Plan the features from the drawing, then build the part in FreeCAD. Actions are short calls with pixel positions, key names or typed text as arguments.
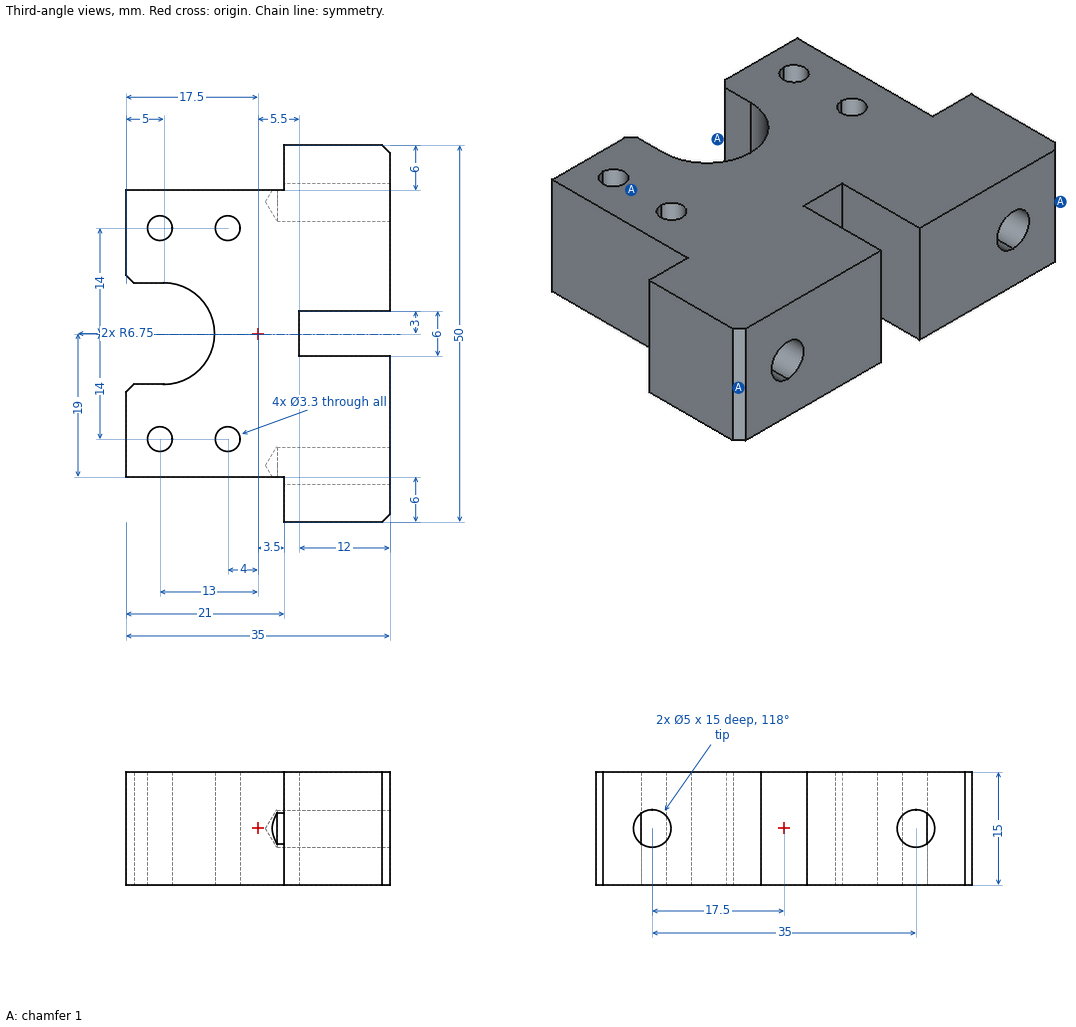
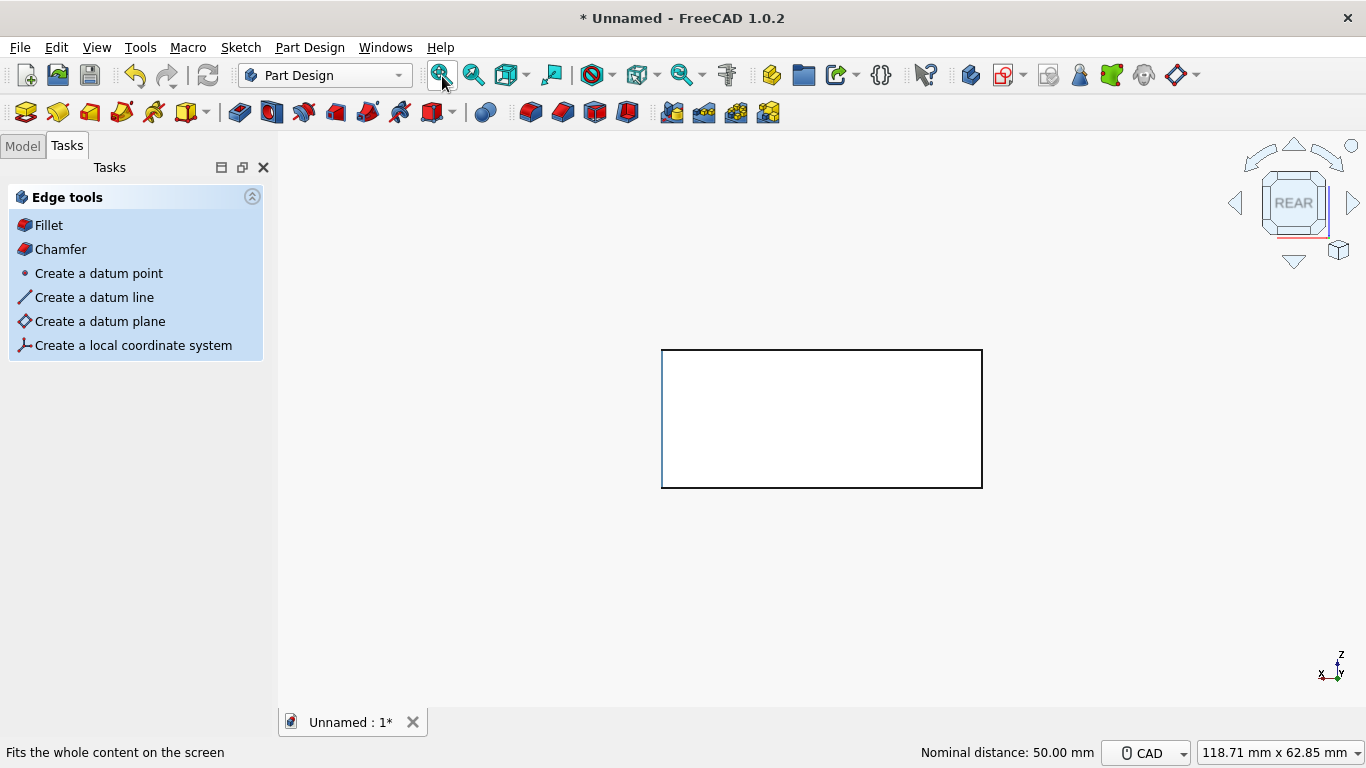
key(6)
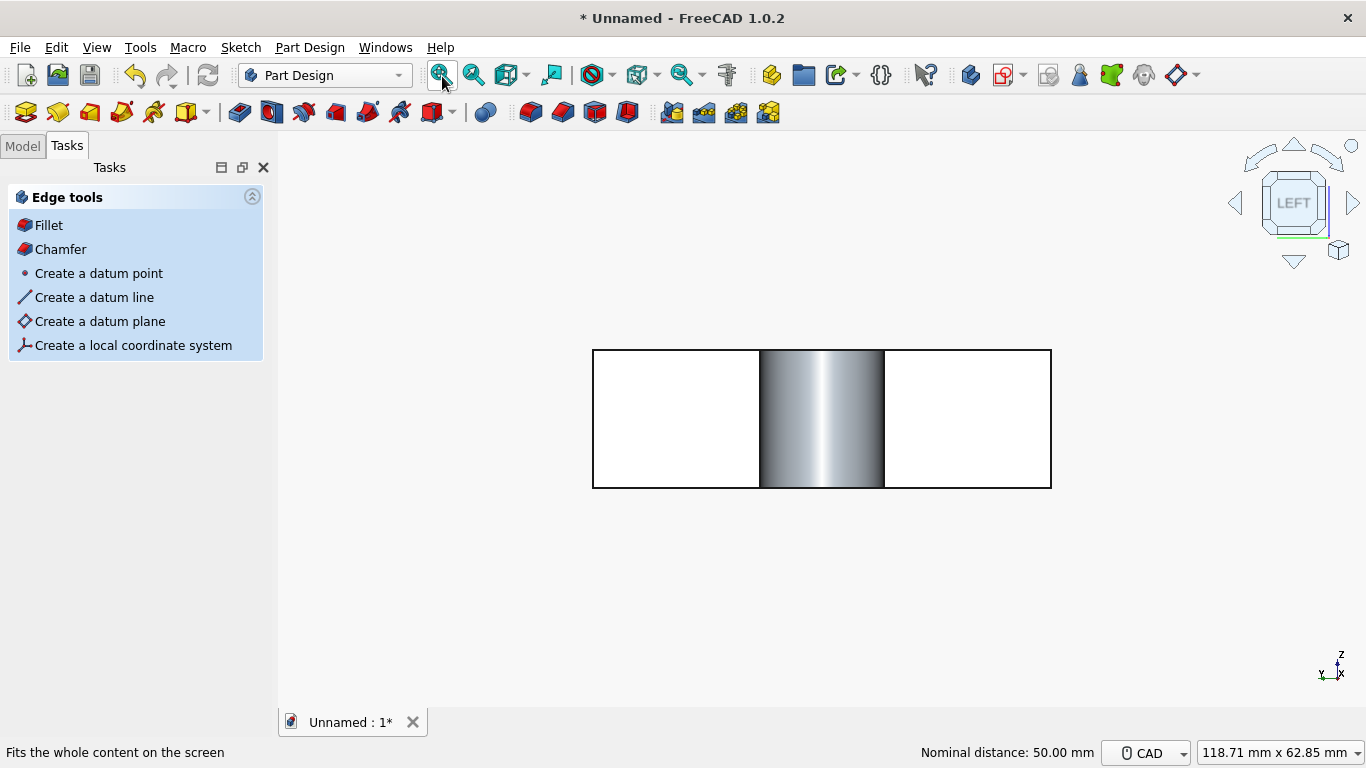
click(442, 76)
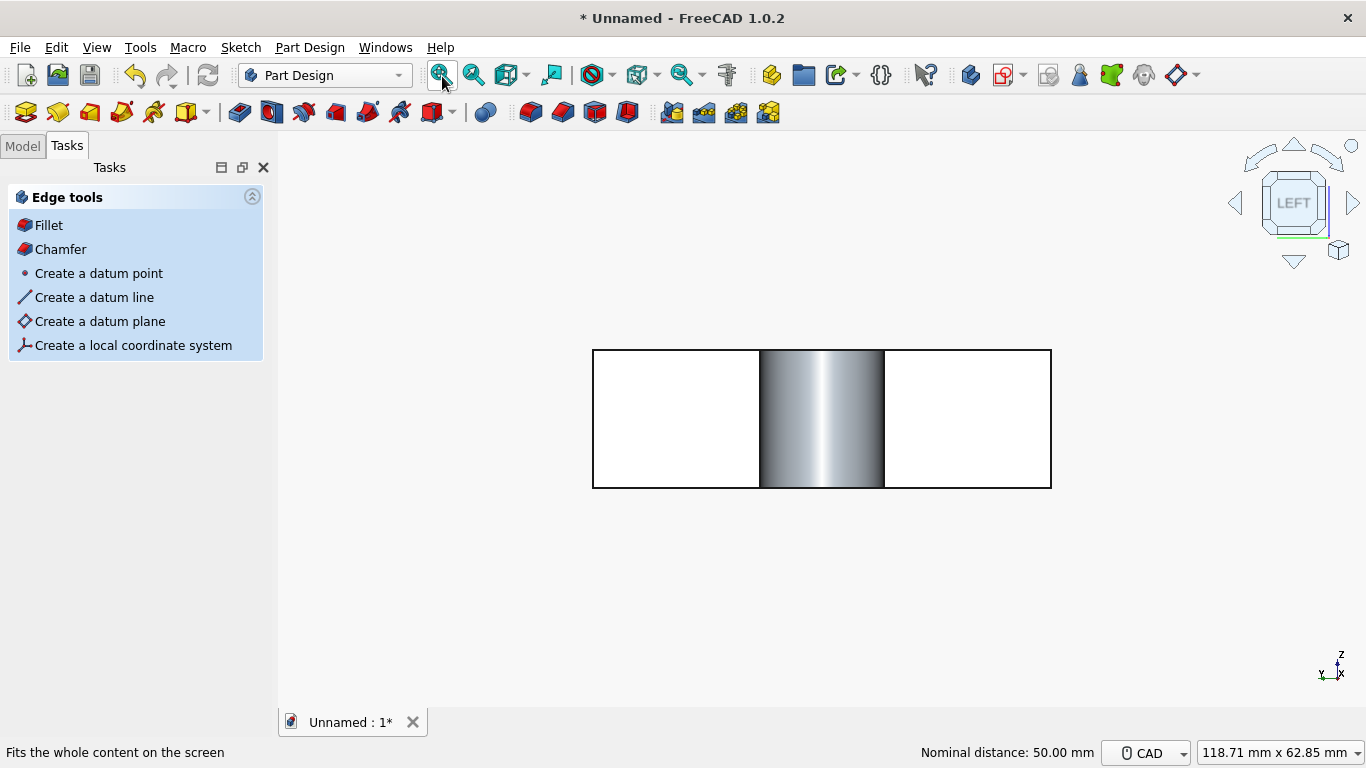
click(884, 418, ctrl)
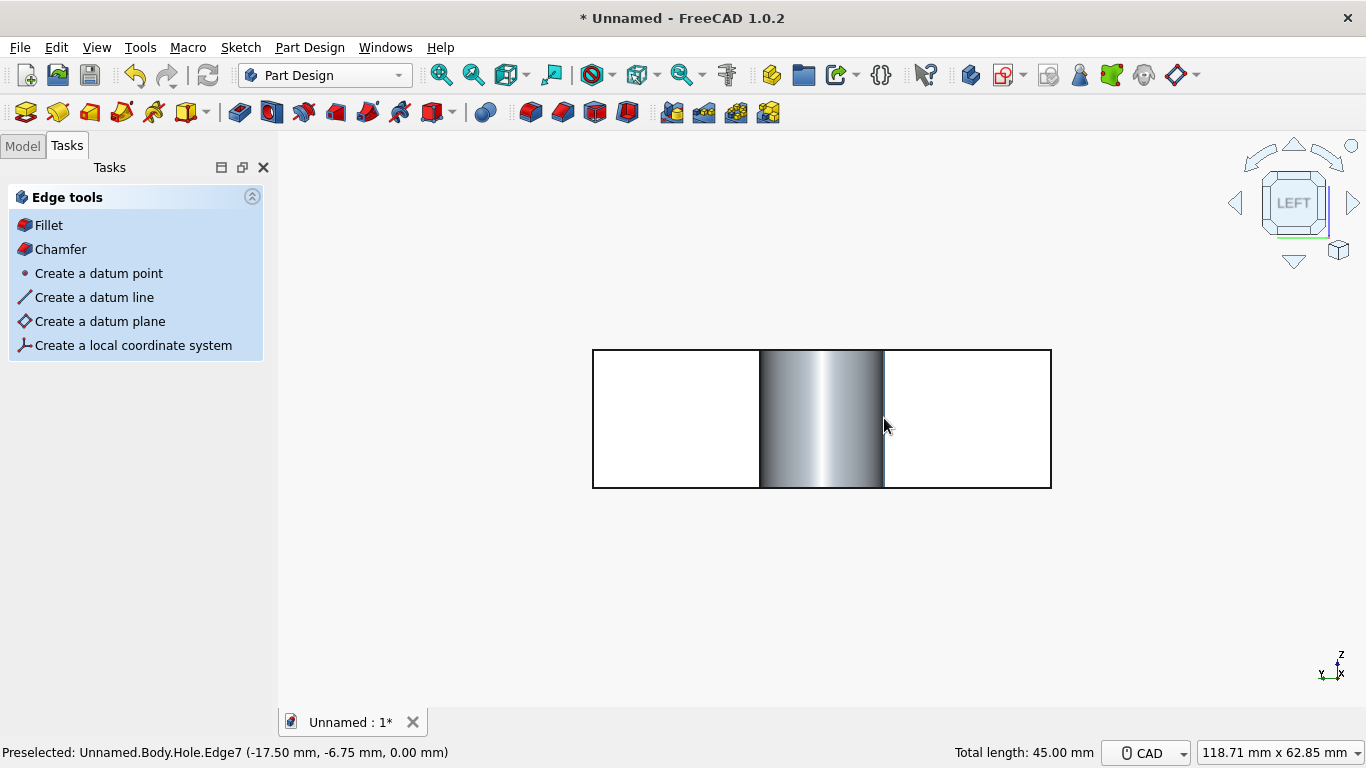
click(760, 418, ctrl)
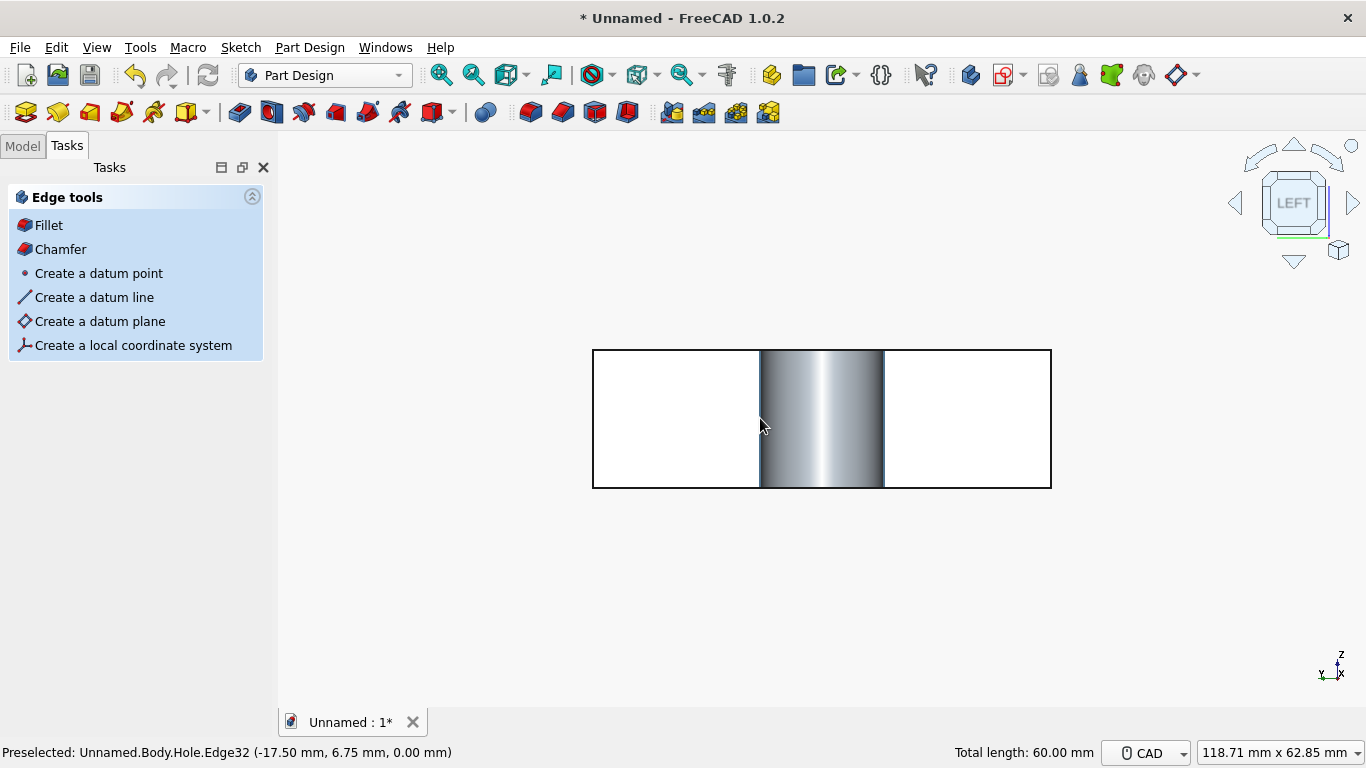
click(564, 112)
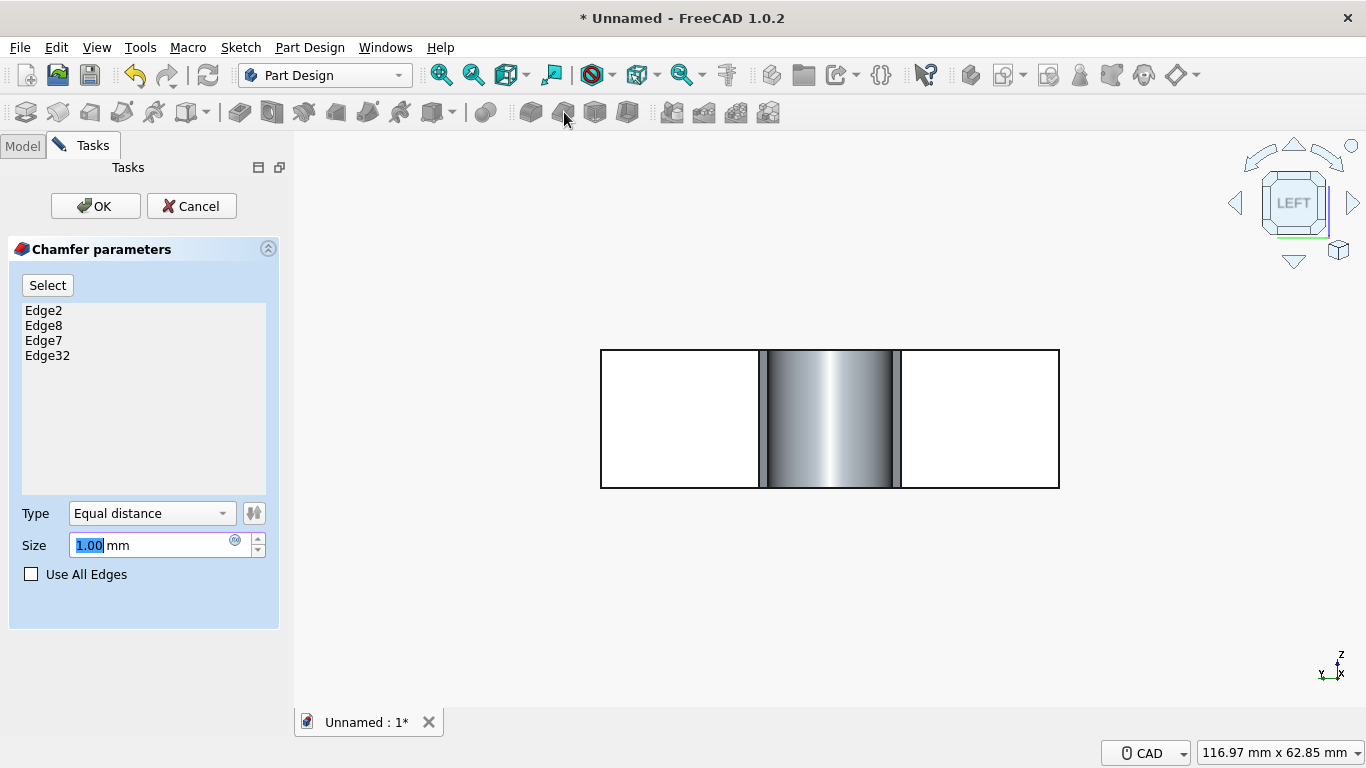
text(1)
key(Tab)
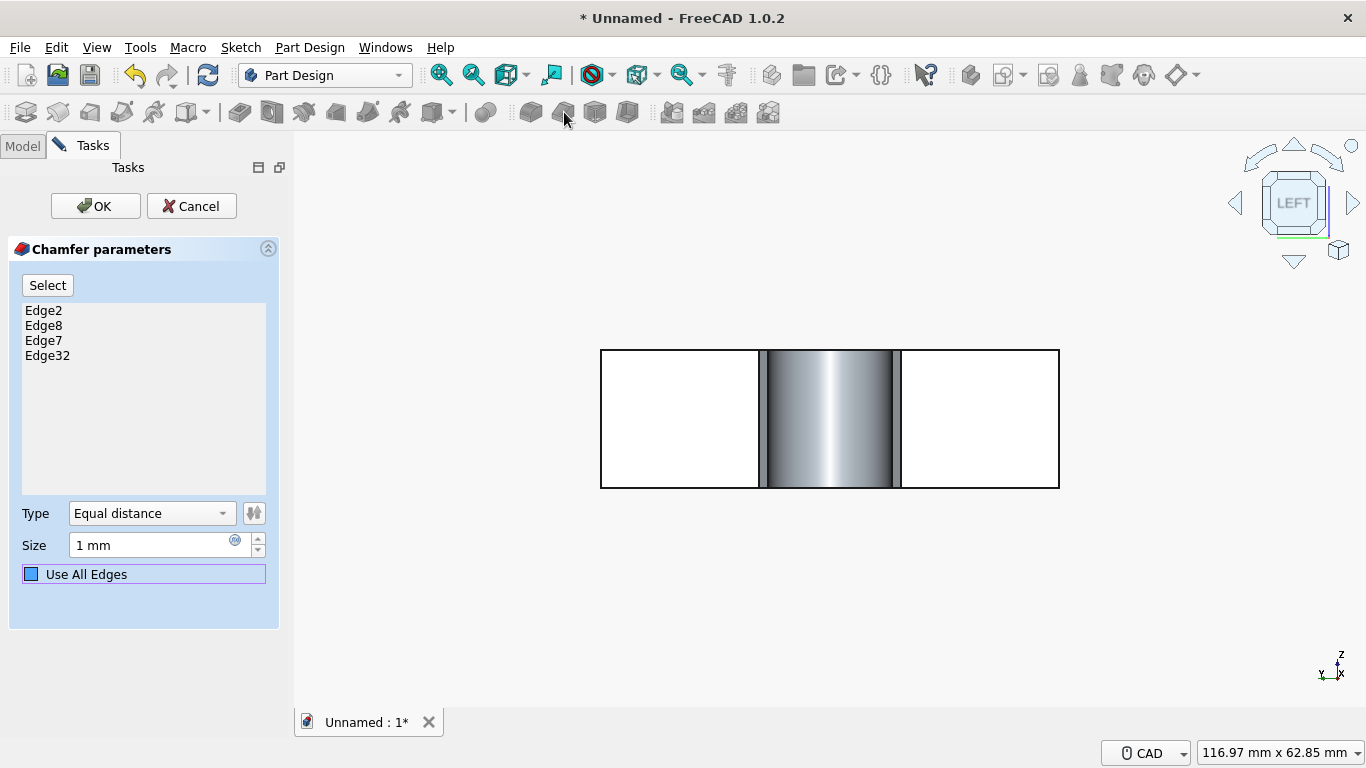
click(96, 206)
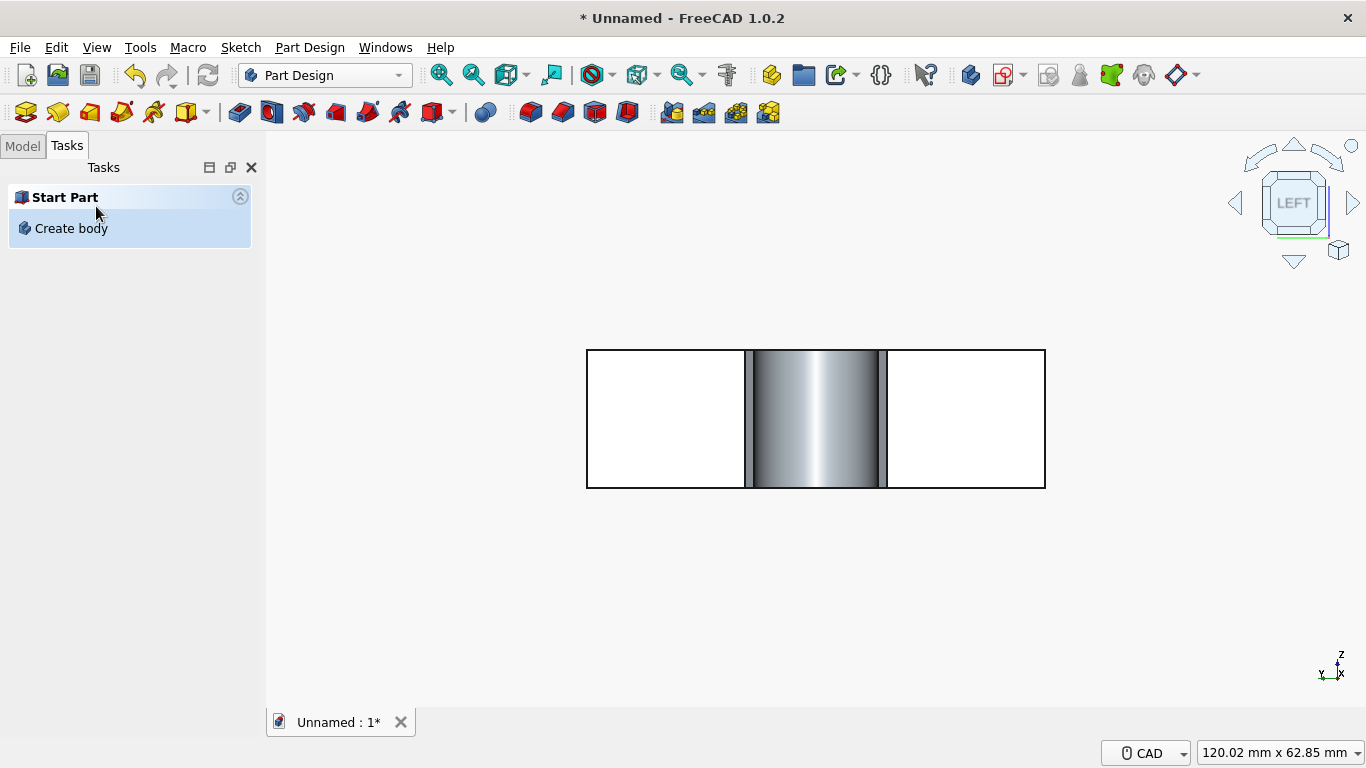
click(442, 76)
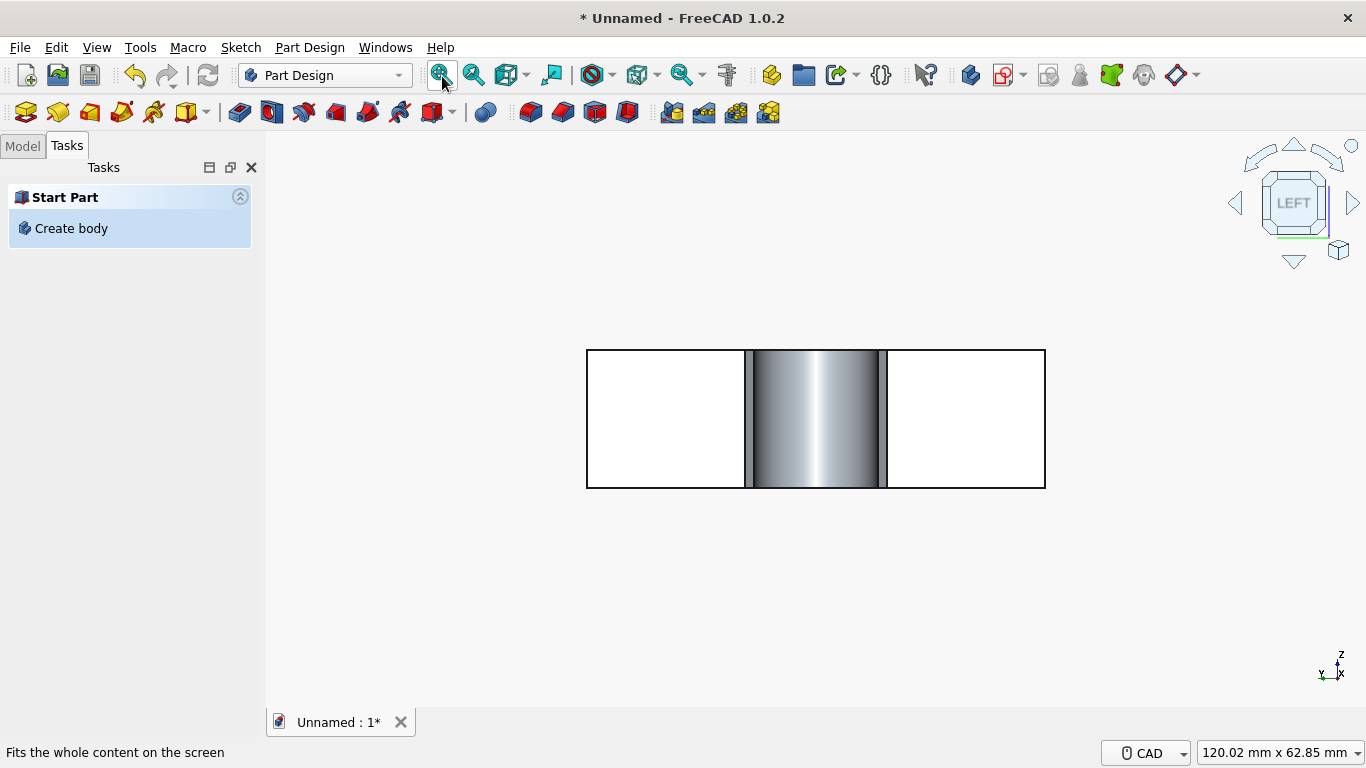
key(0)